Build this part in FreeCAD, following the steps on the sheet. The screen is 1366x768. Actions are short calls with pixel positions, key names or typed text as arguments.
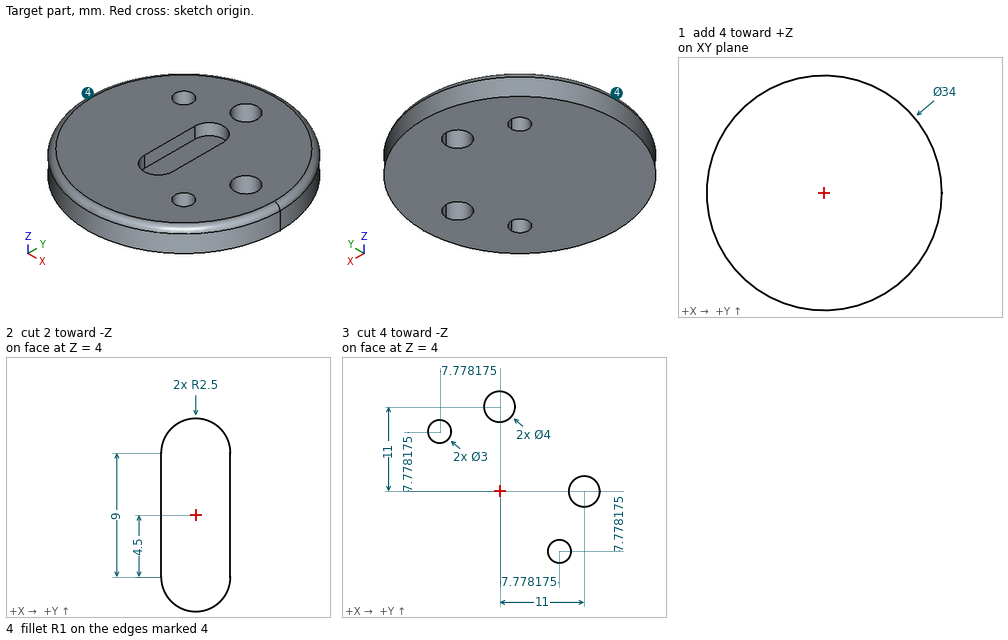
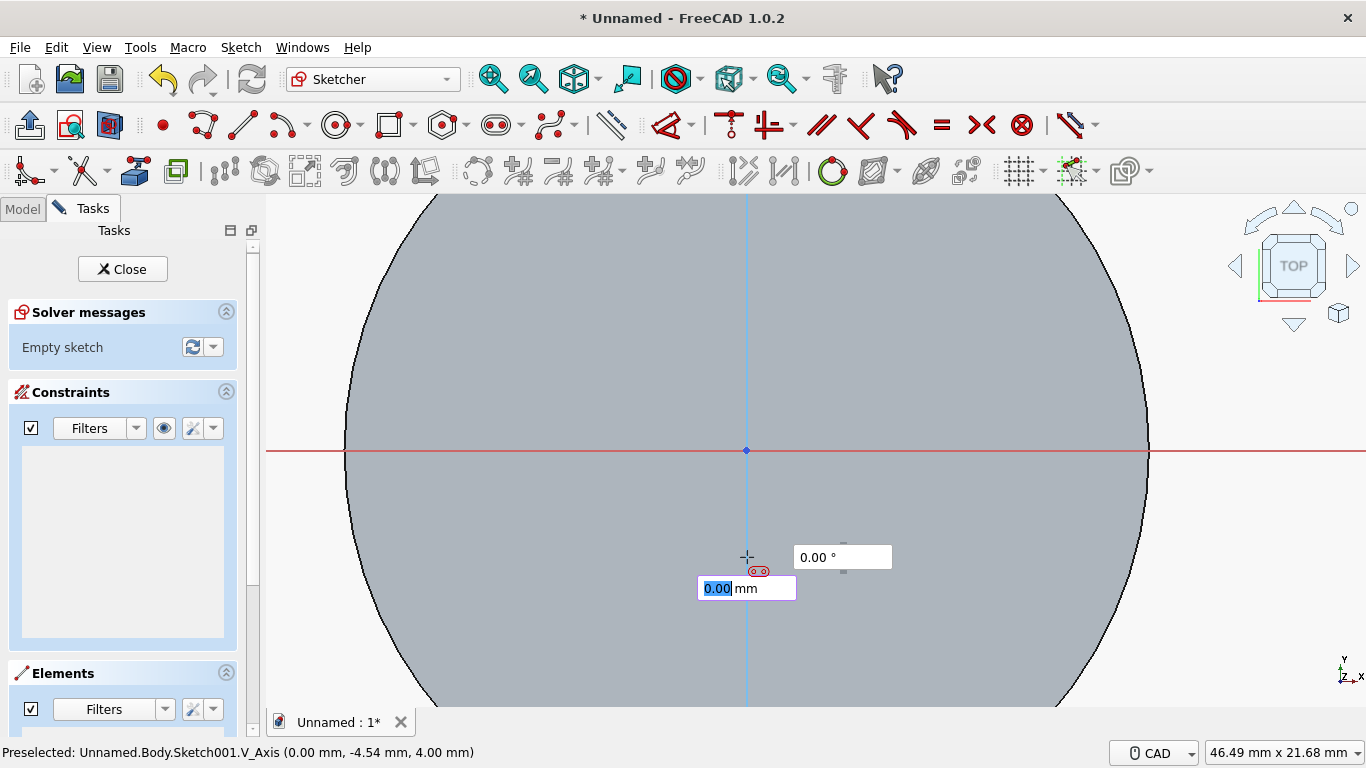
click(756, 344)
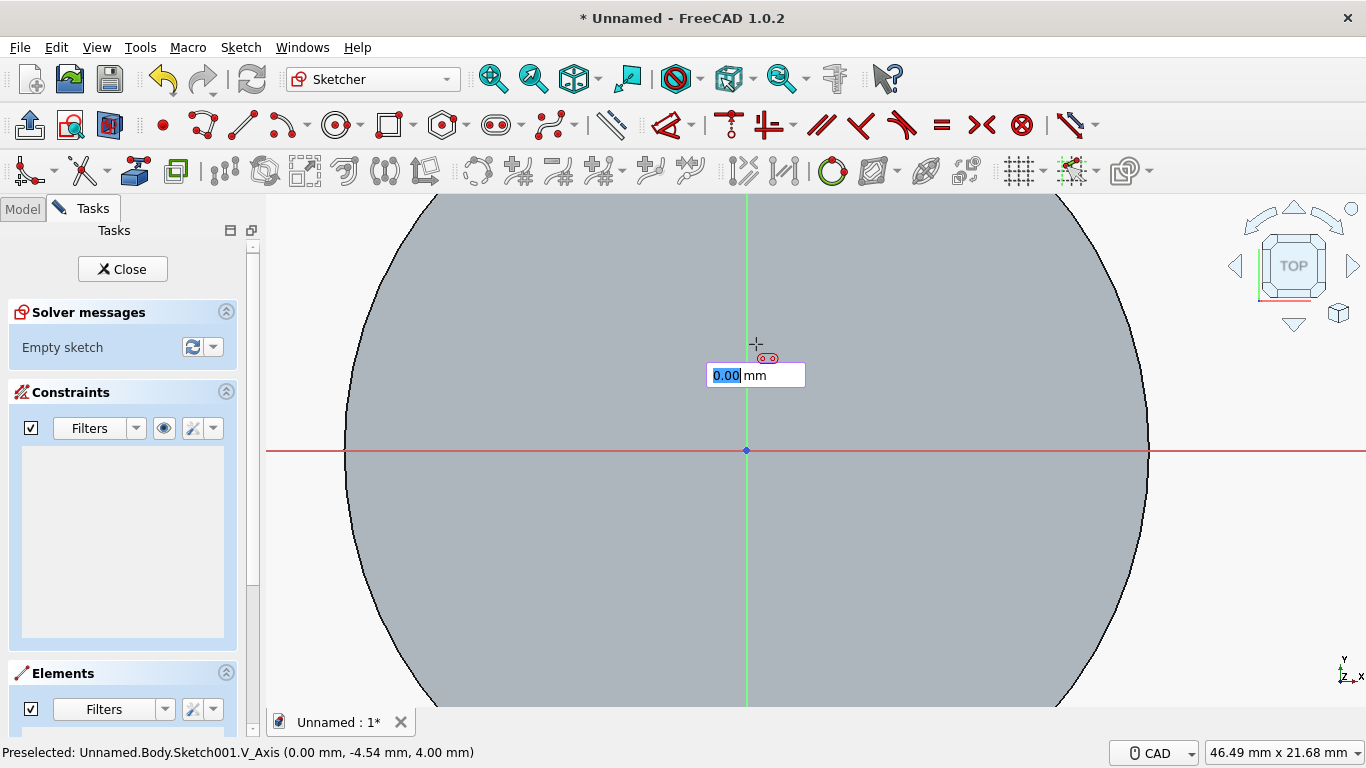
click(806, 482)
key(Escape)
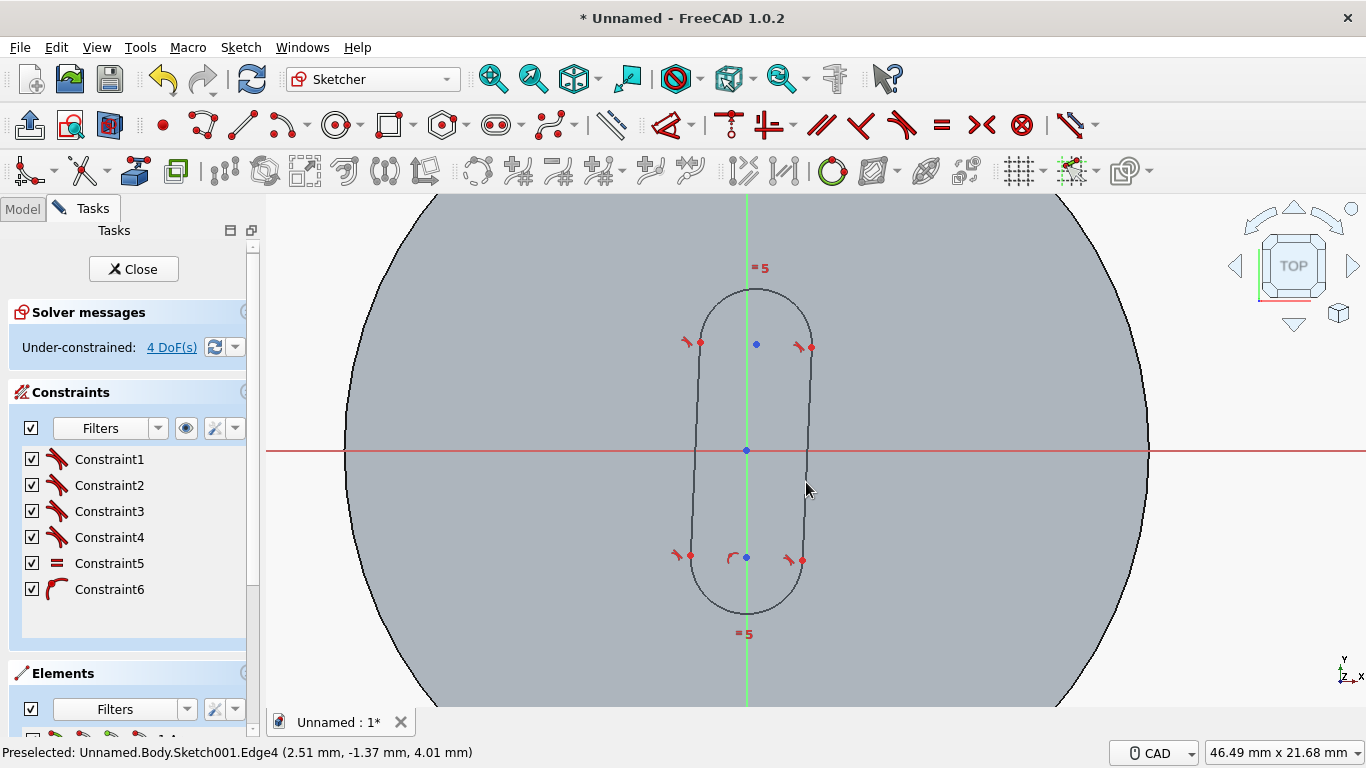
click(694, 492)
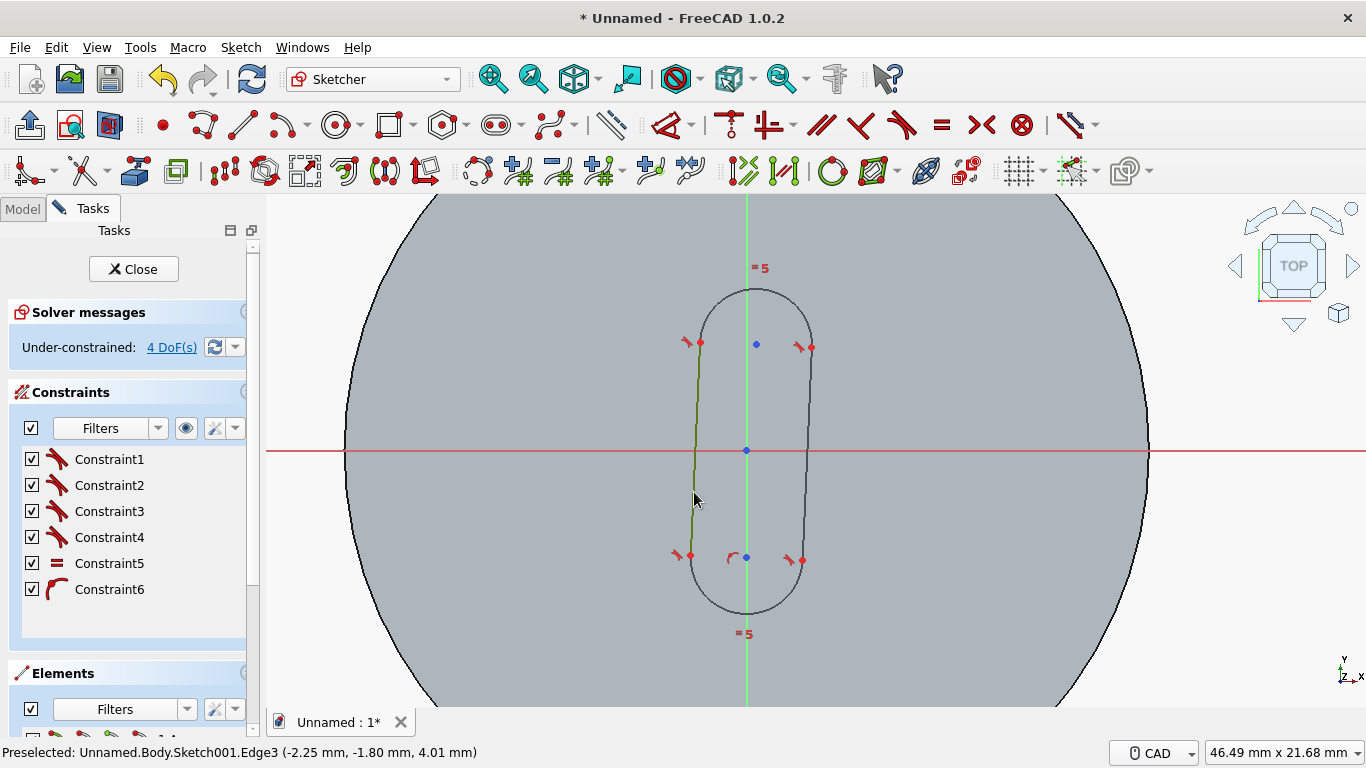
key(v)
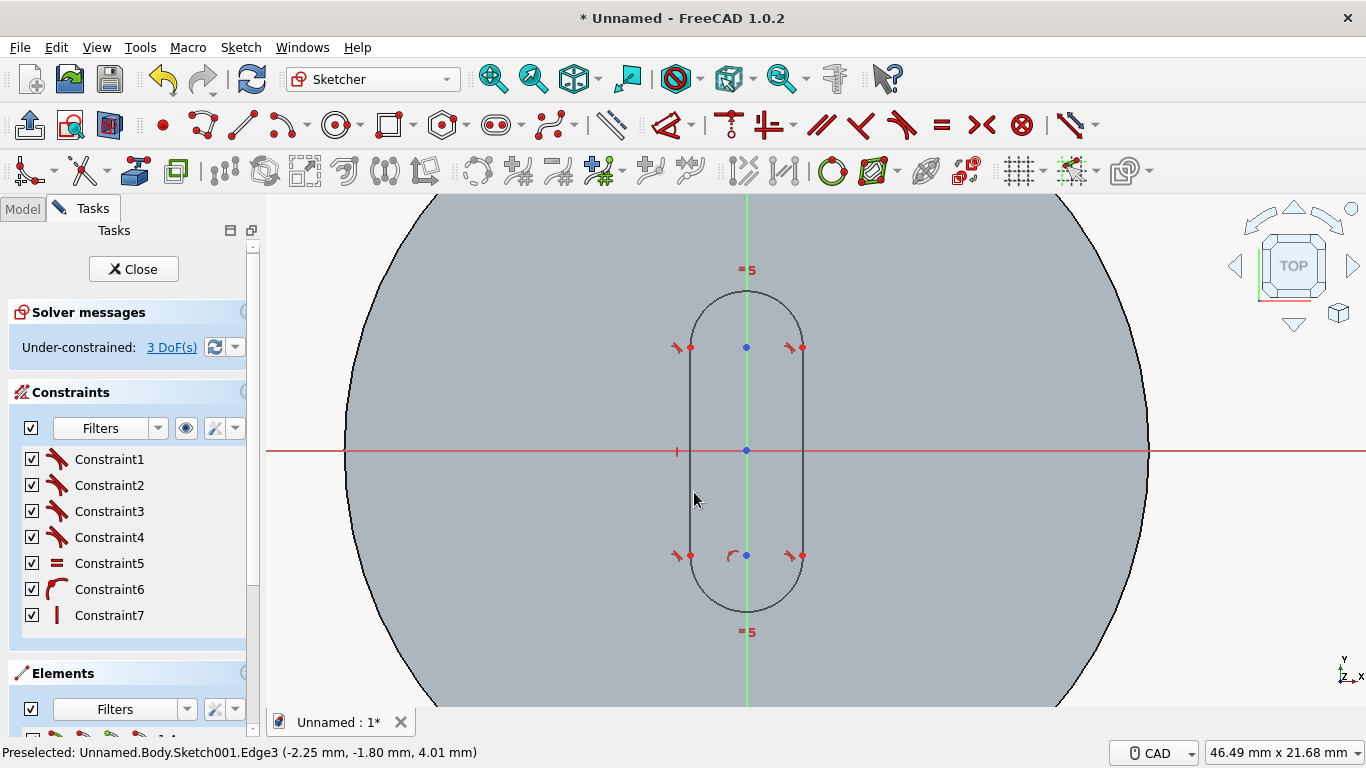
click(666, 126)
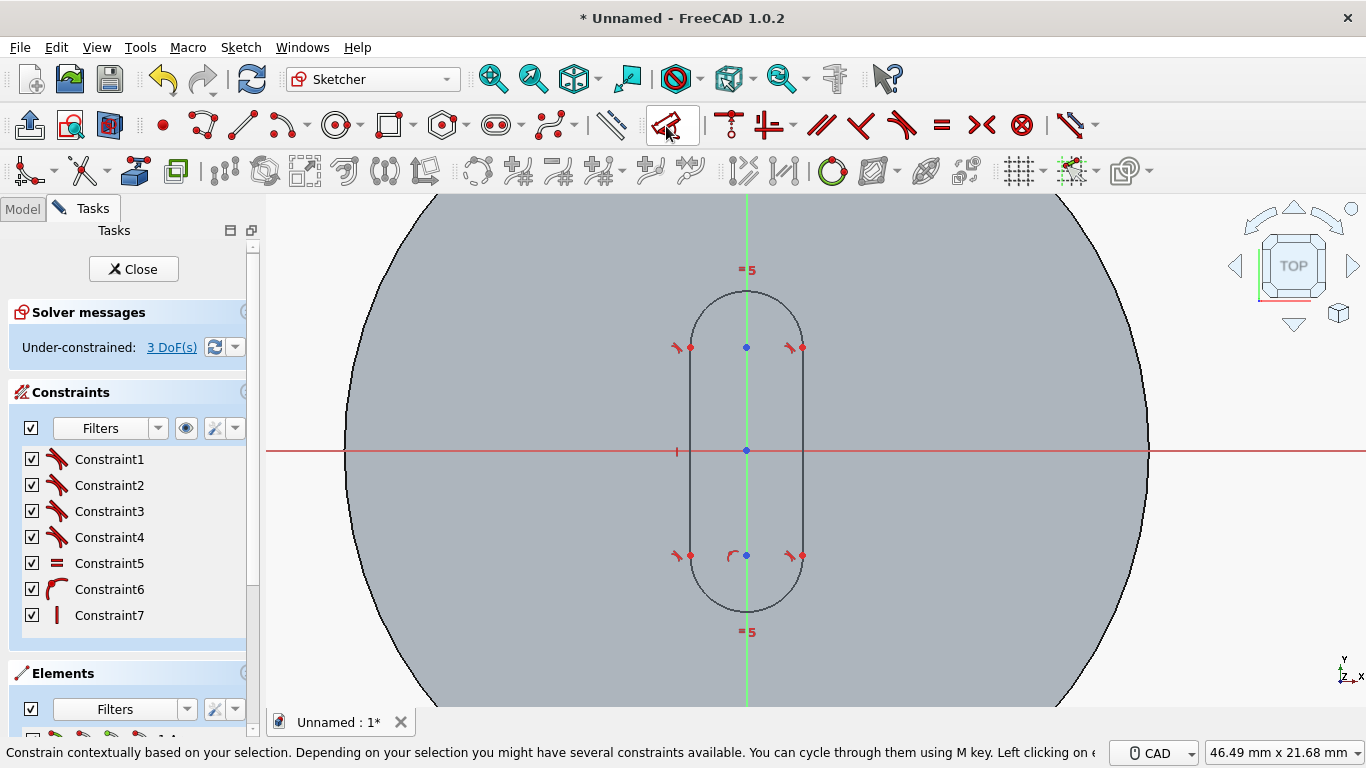
click(714, 601)
click(695, 627)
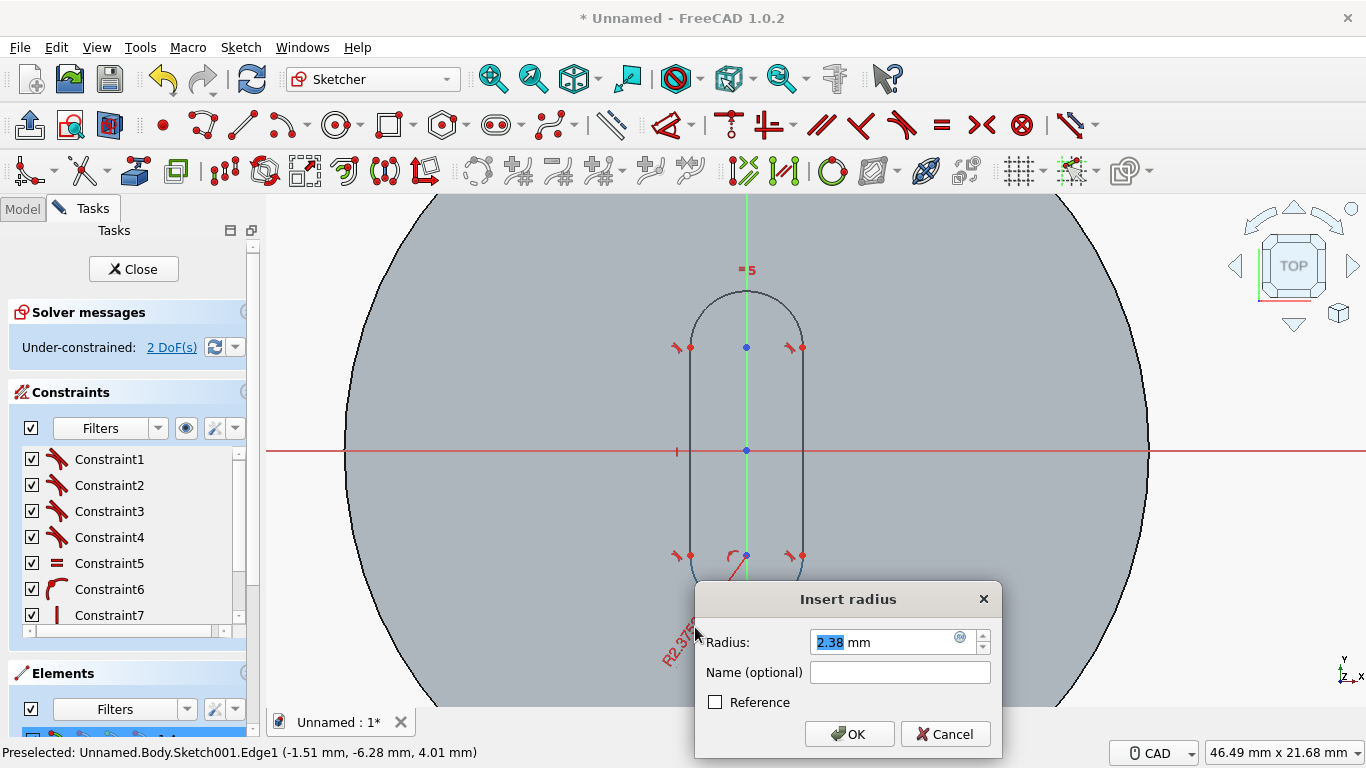
text(2.5)
key(Return)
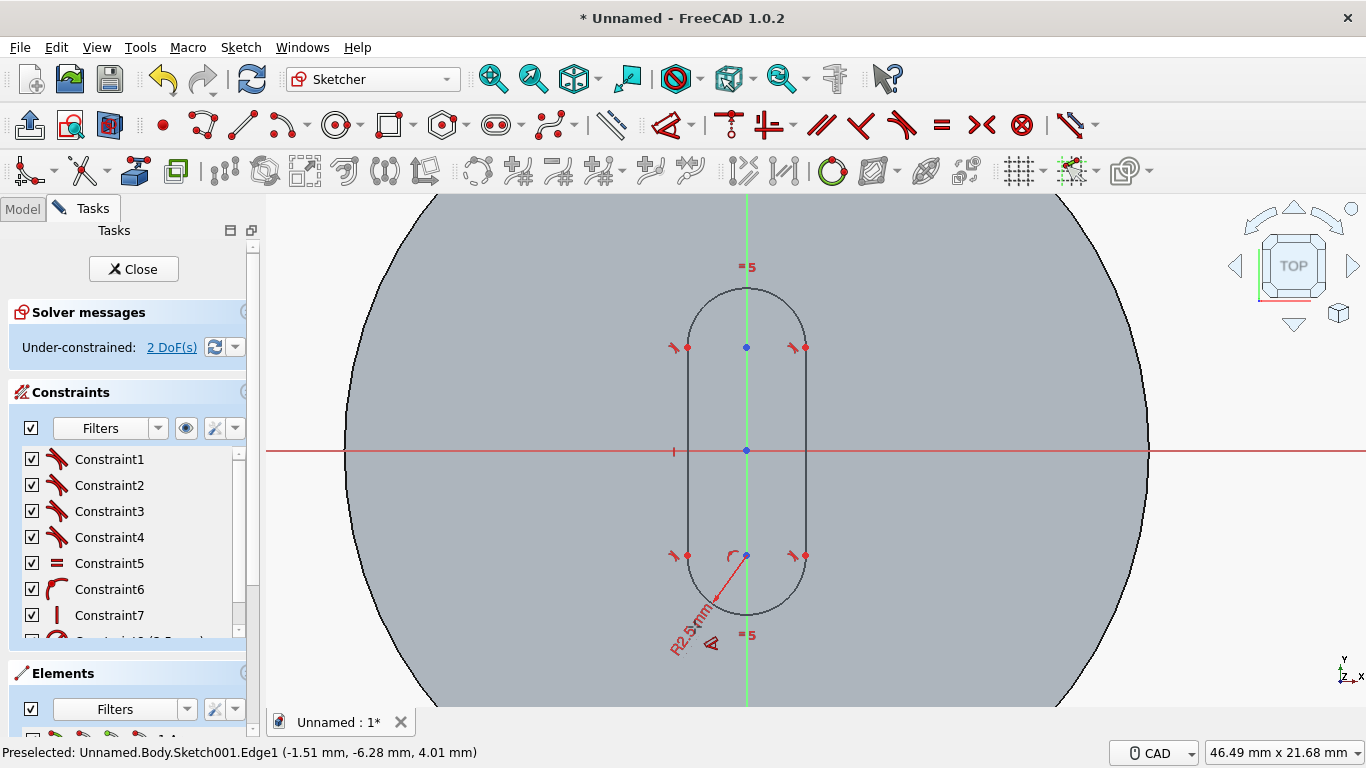
click(688, 493)
click(654, 404)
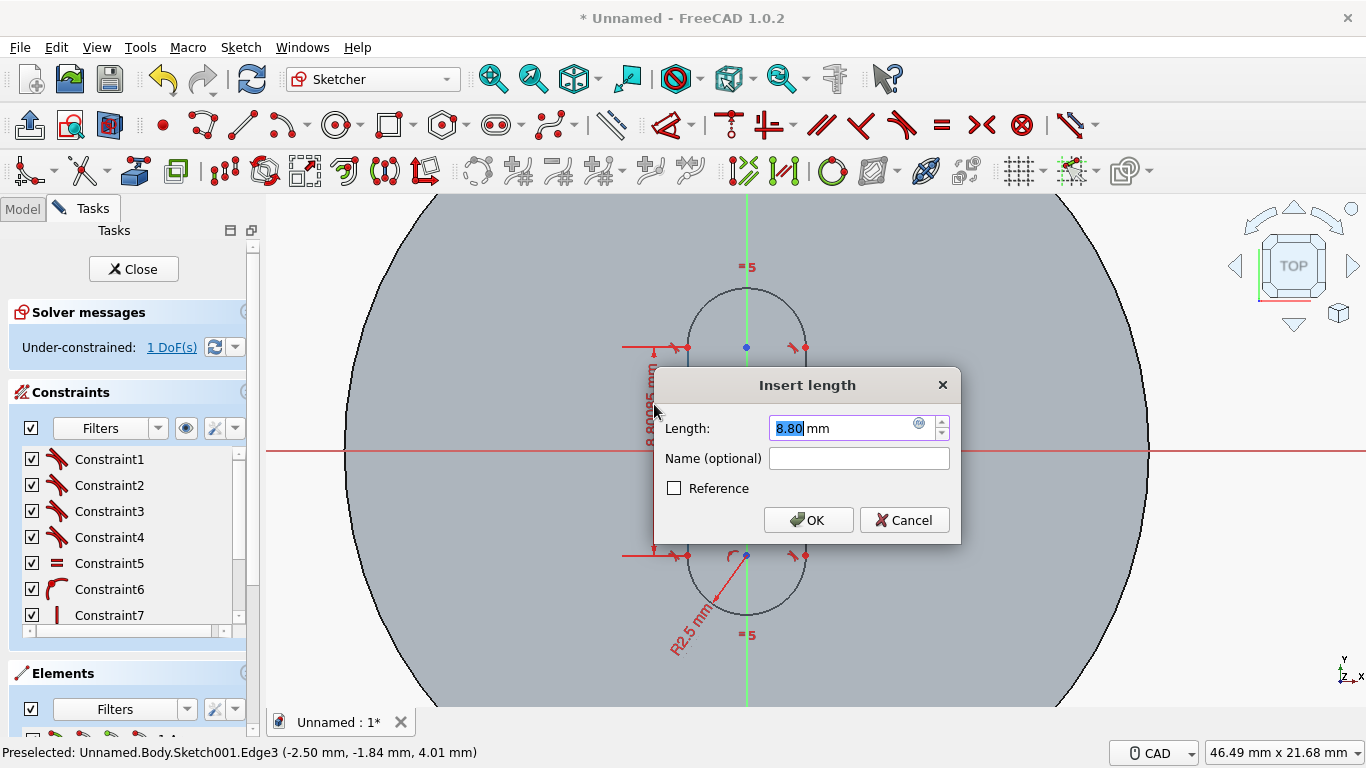
text(9)
key(Return)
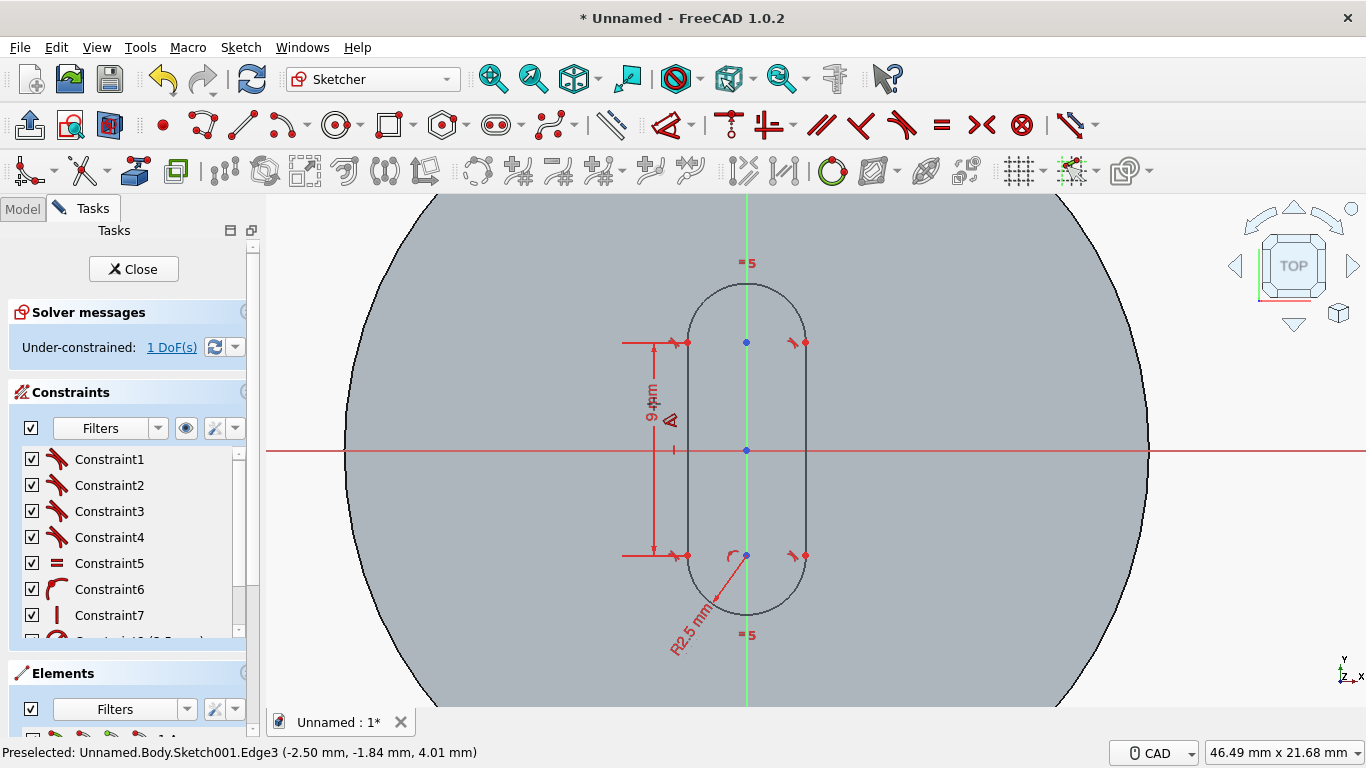
click(688, 556)
click(654, 503)